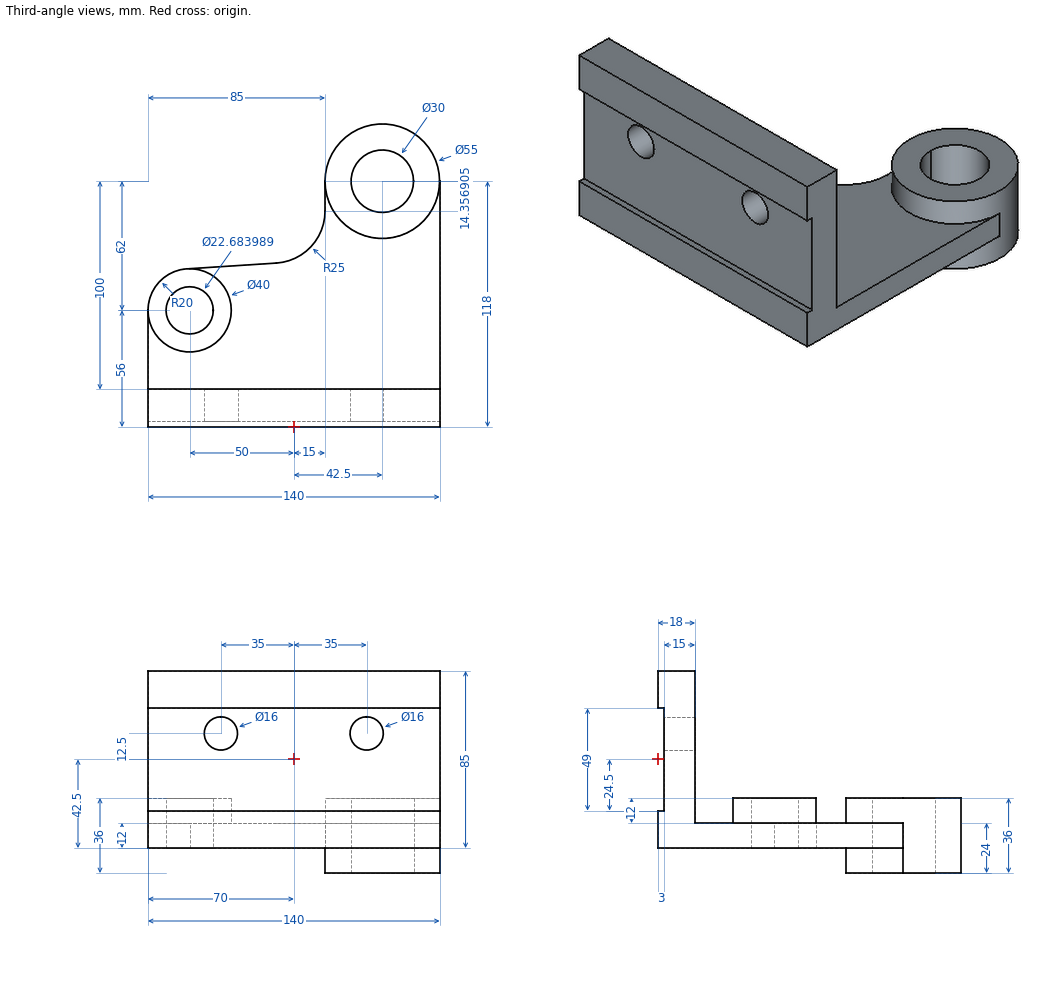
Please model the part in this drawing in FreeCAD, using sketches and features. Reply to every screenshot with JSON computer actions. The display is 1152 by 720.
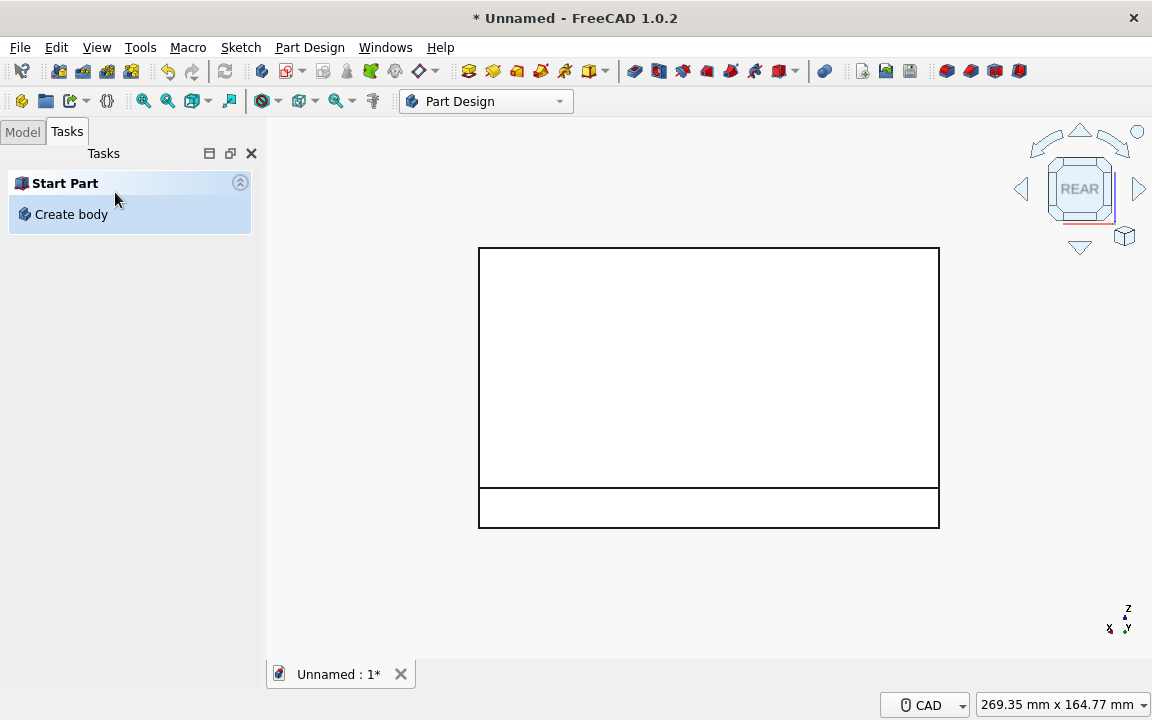
{"action": "key", "text": "0"}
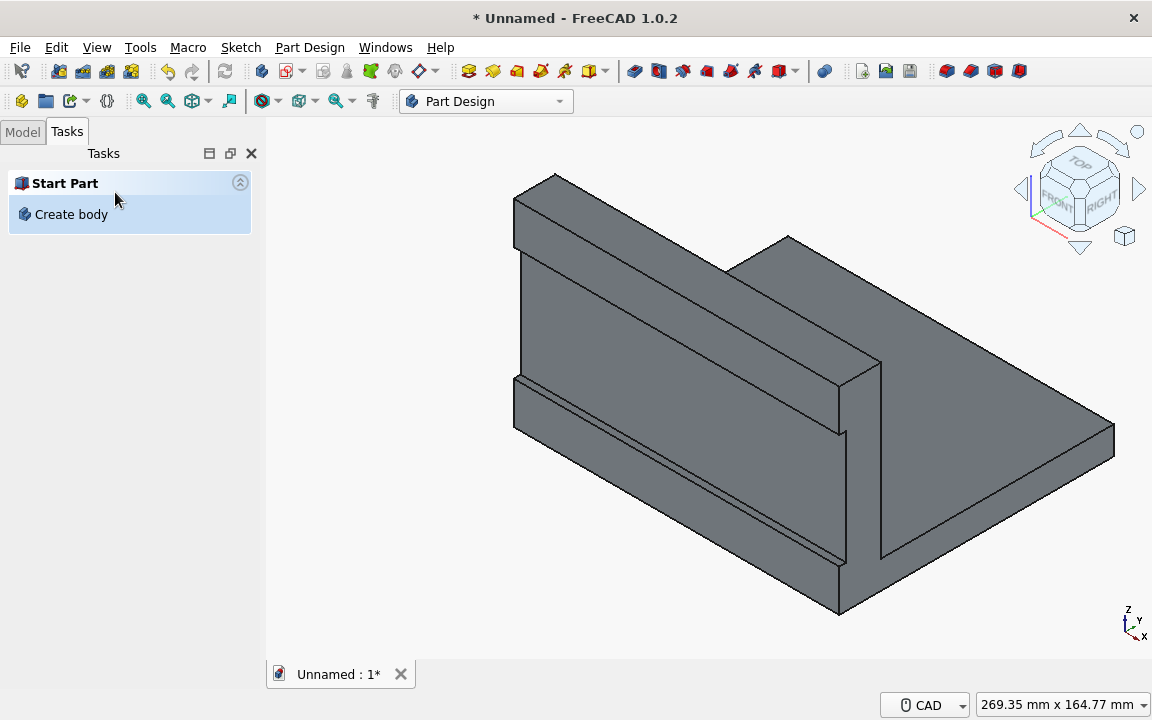
{"action": "key", "text": "v f"}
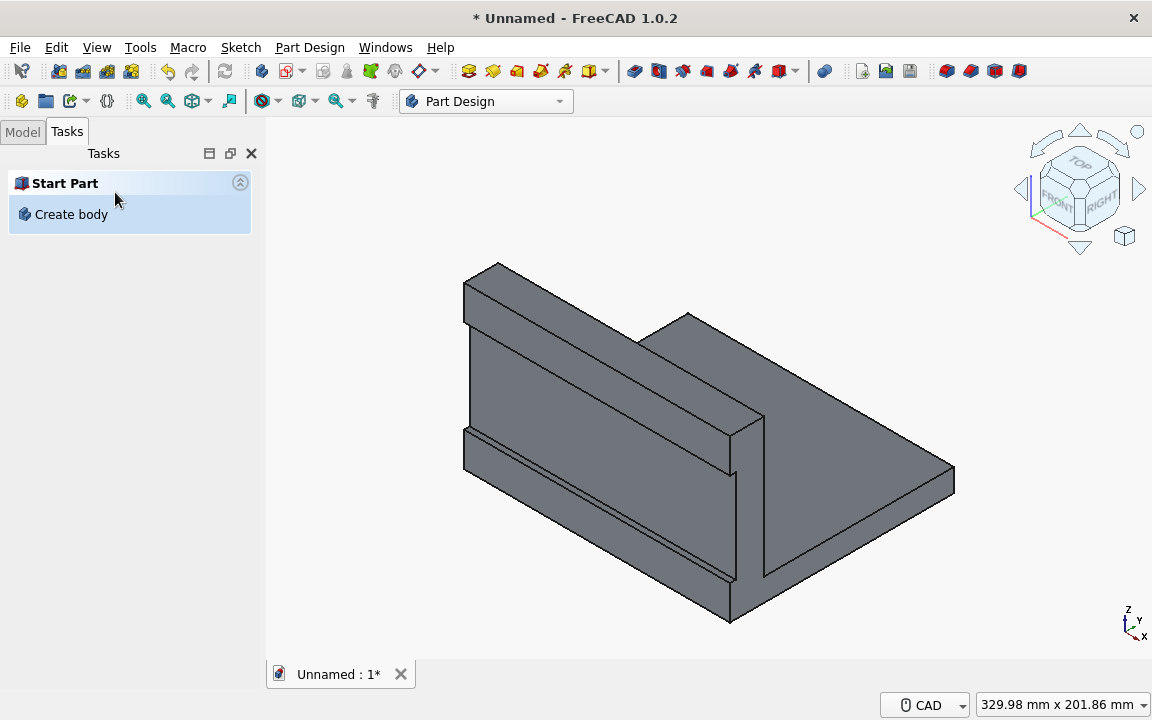
{"action": "left_click", "coordinate": [791, 450]}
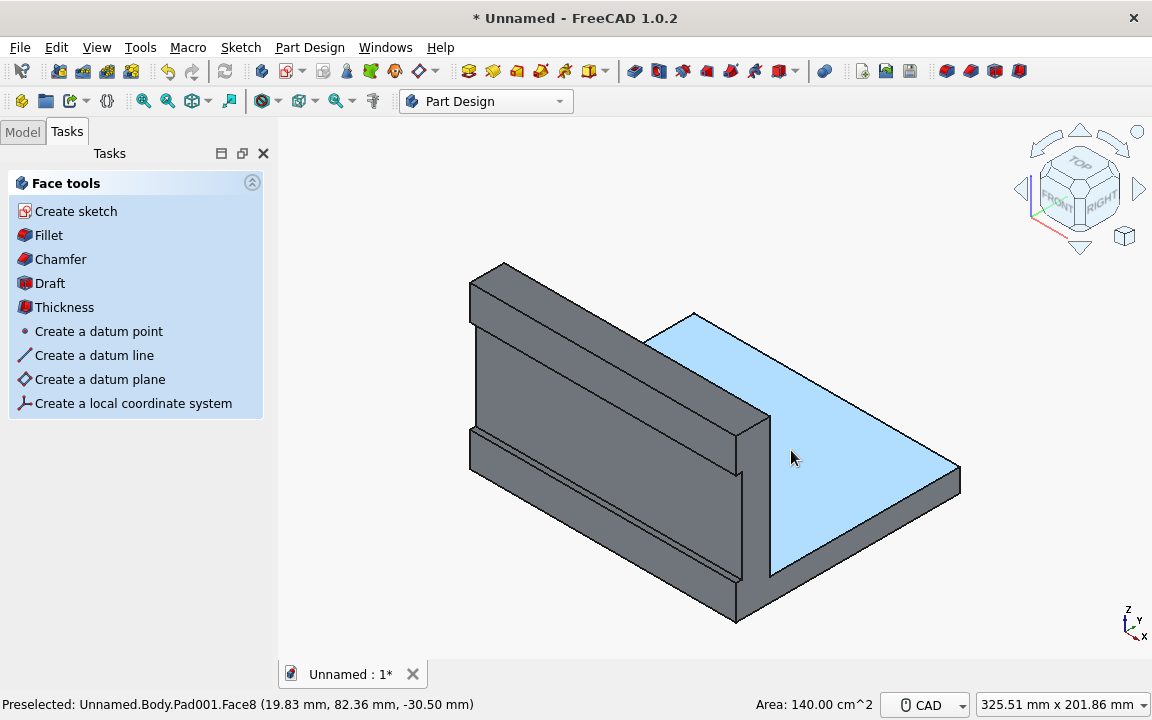
{"action": "left_click", "coordinate": [286, 72]}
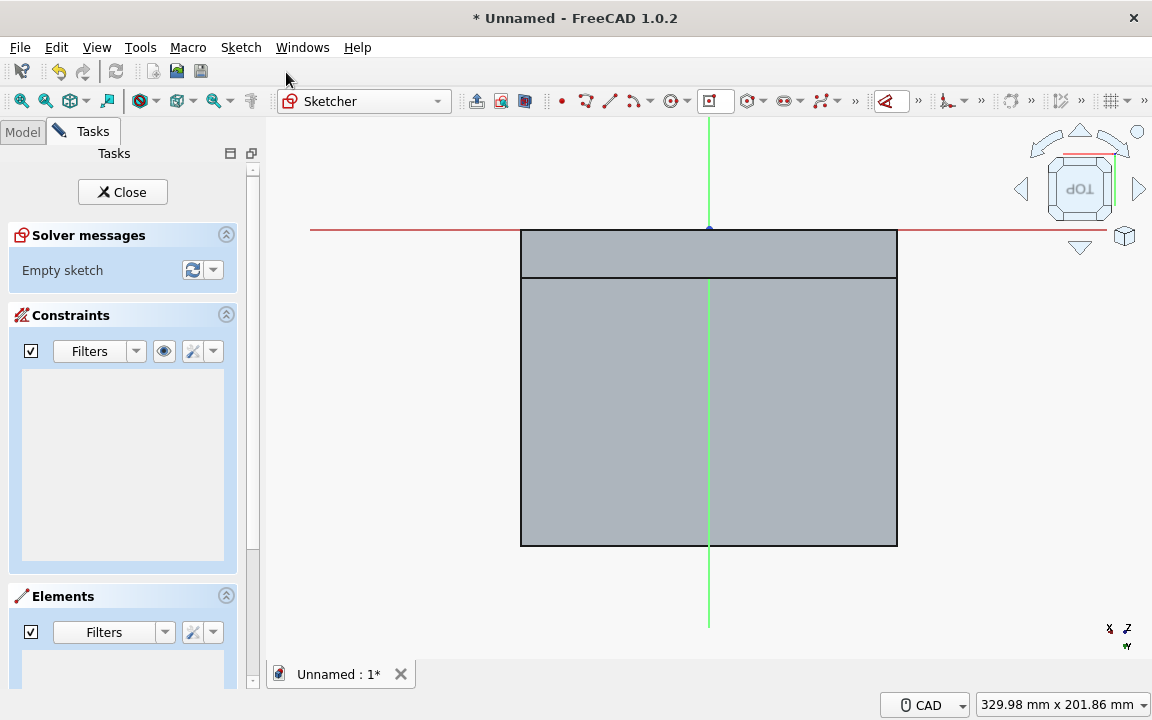
{"action": "left_click", "coordinate": [526, 102]}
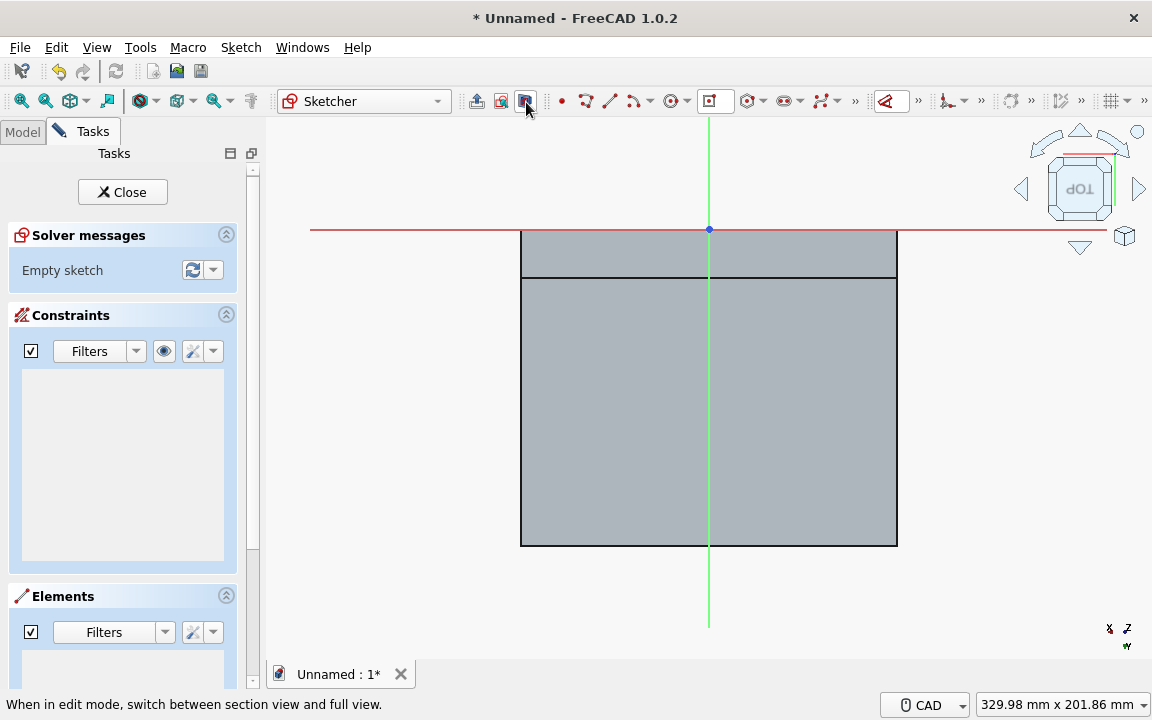
{"action": "scroll", "coordinate": [987, 263], "scroll_direction": "up", "scroll_amount": 3}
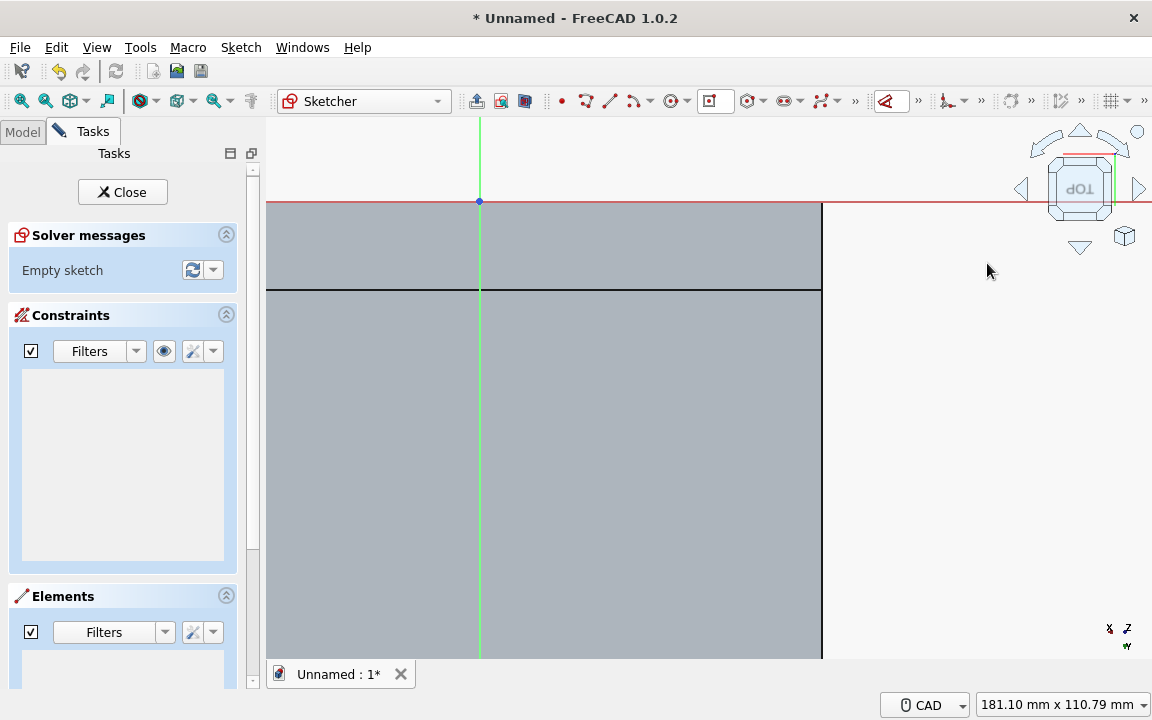
{"action": "key", "text": "g c"}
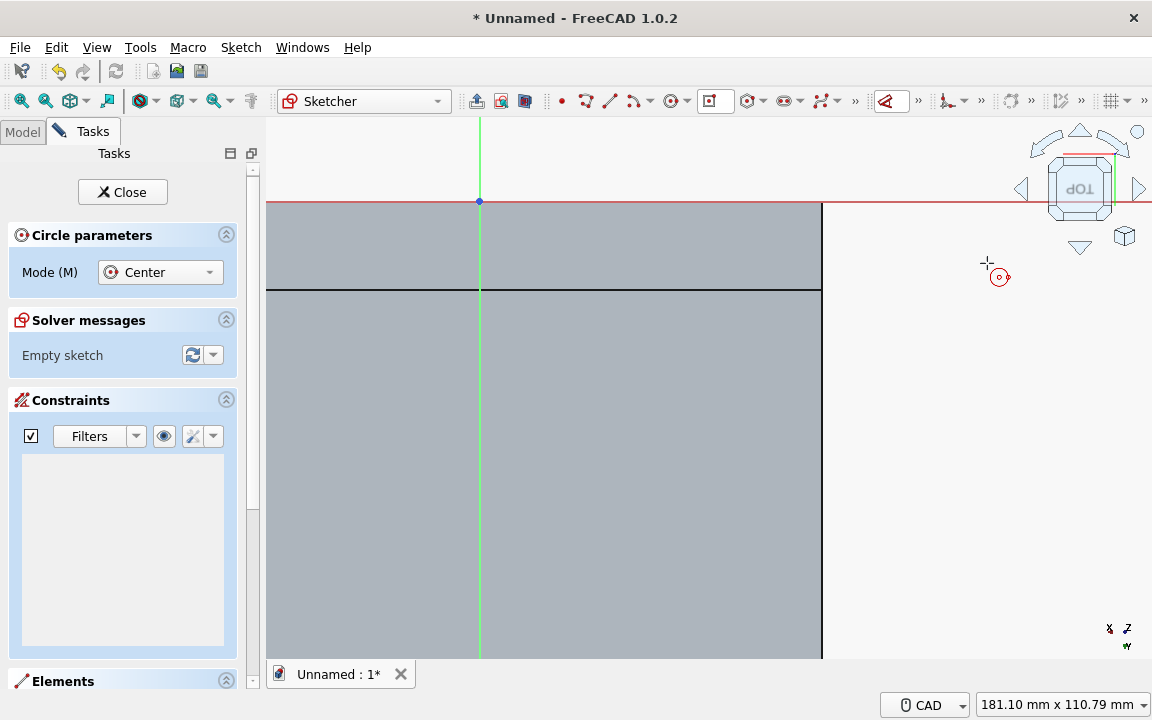
{"action": "left_click", "coordinate": [724, 476]}
{"action": "left_click", "coordinate": [794, 407]}
{"action": "key", "text": "Escape"}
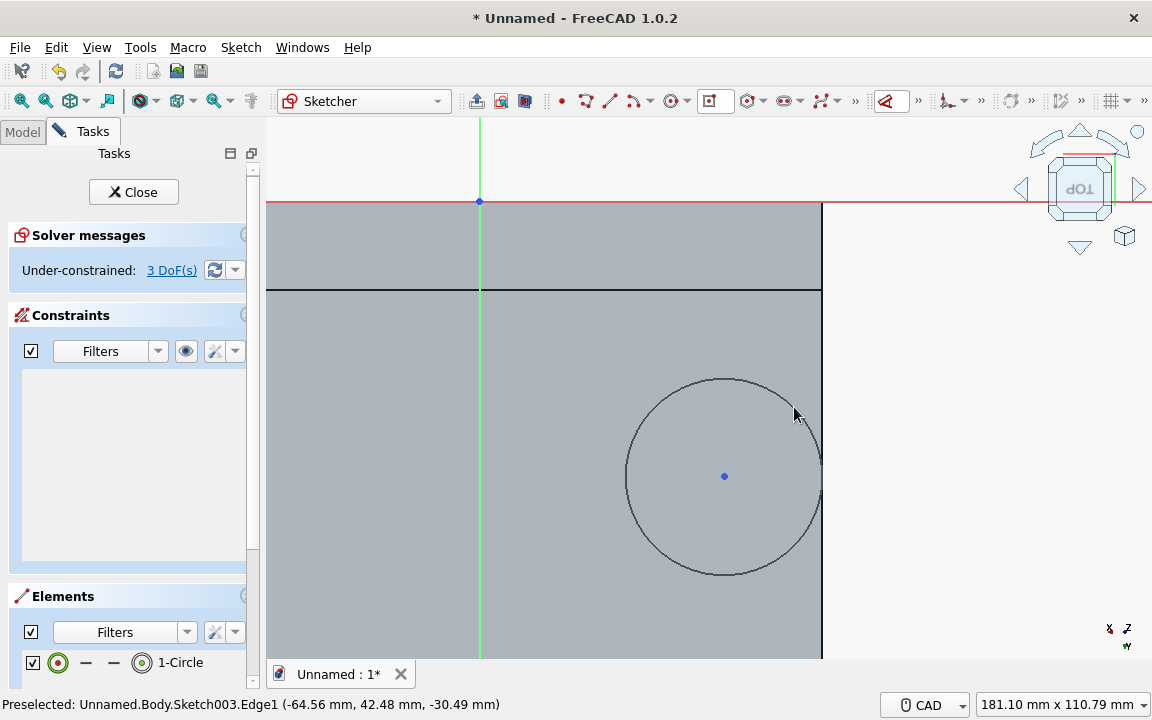
{"action": "left_click", "coordinate": [793, 407]}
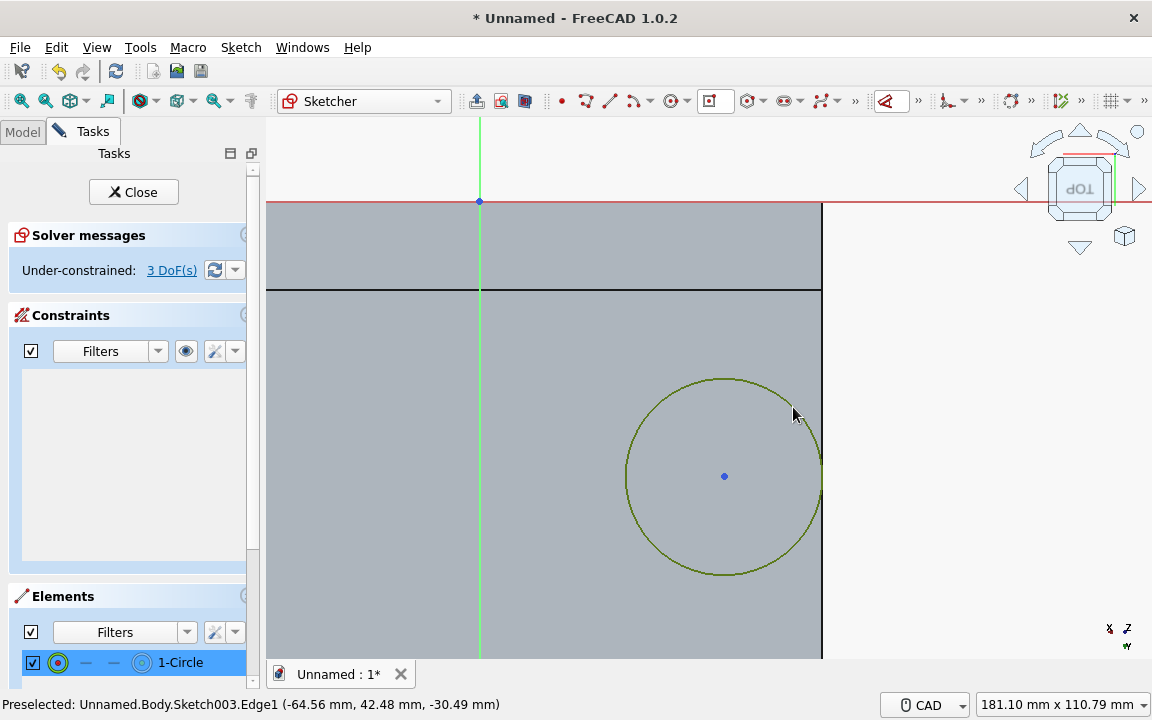
{"action": "key", "text": "k o"}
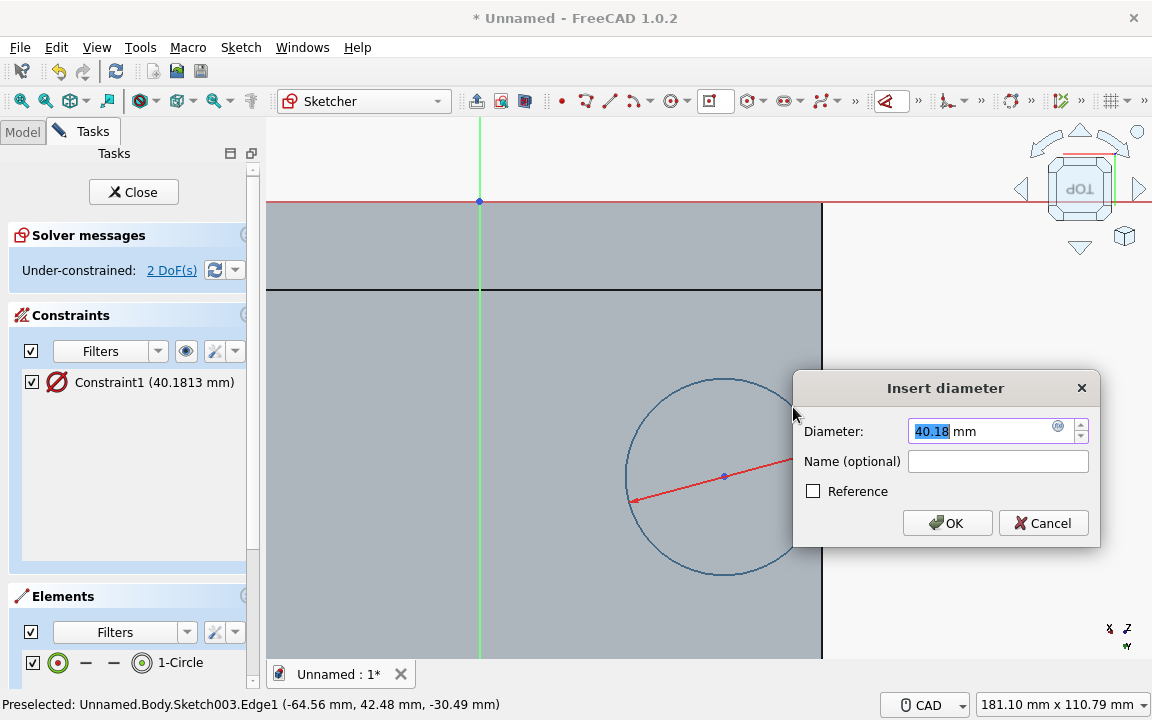
{"action": "type", "text": "40"}
{"action": "key", "text": "Return"}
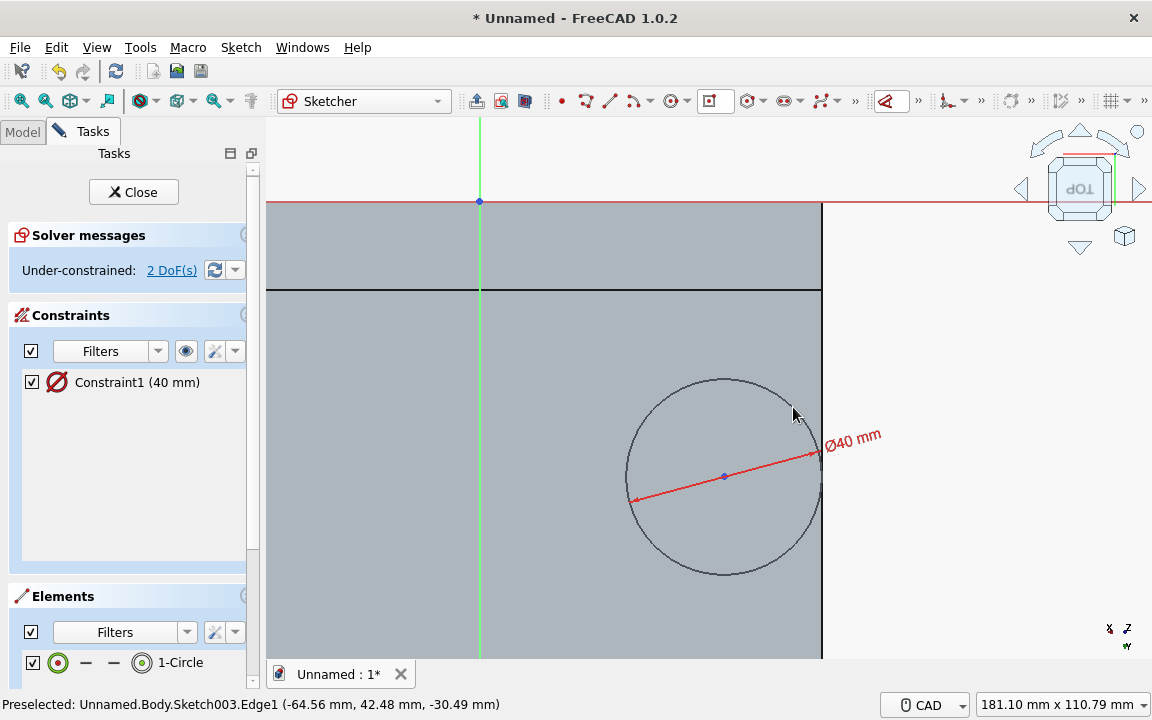
{"action": "left_click", "coordinate": [724, 477]}